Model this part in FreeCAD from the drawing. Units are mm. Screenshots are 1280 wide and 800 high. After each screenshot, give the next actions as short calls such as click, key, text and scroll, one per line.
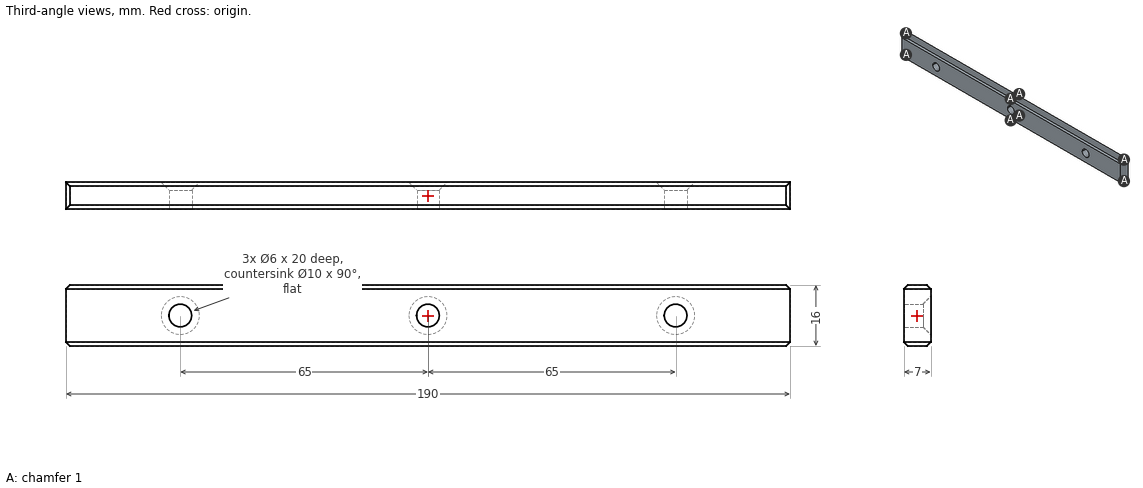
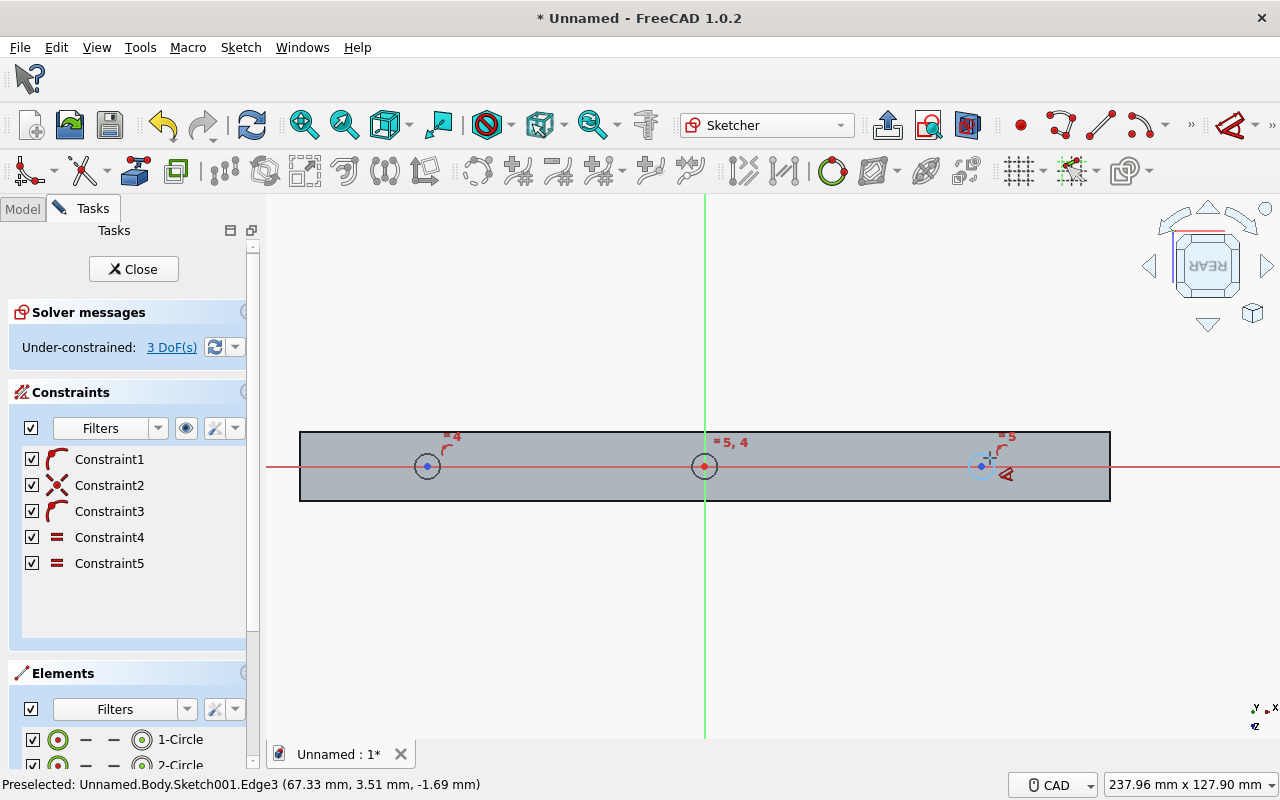
scroll(436, 458, up, 3)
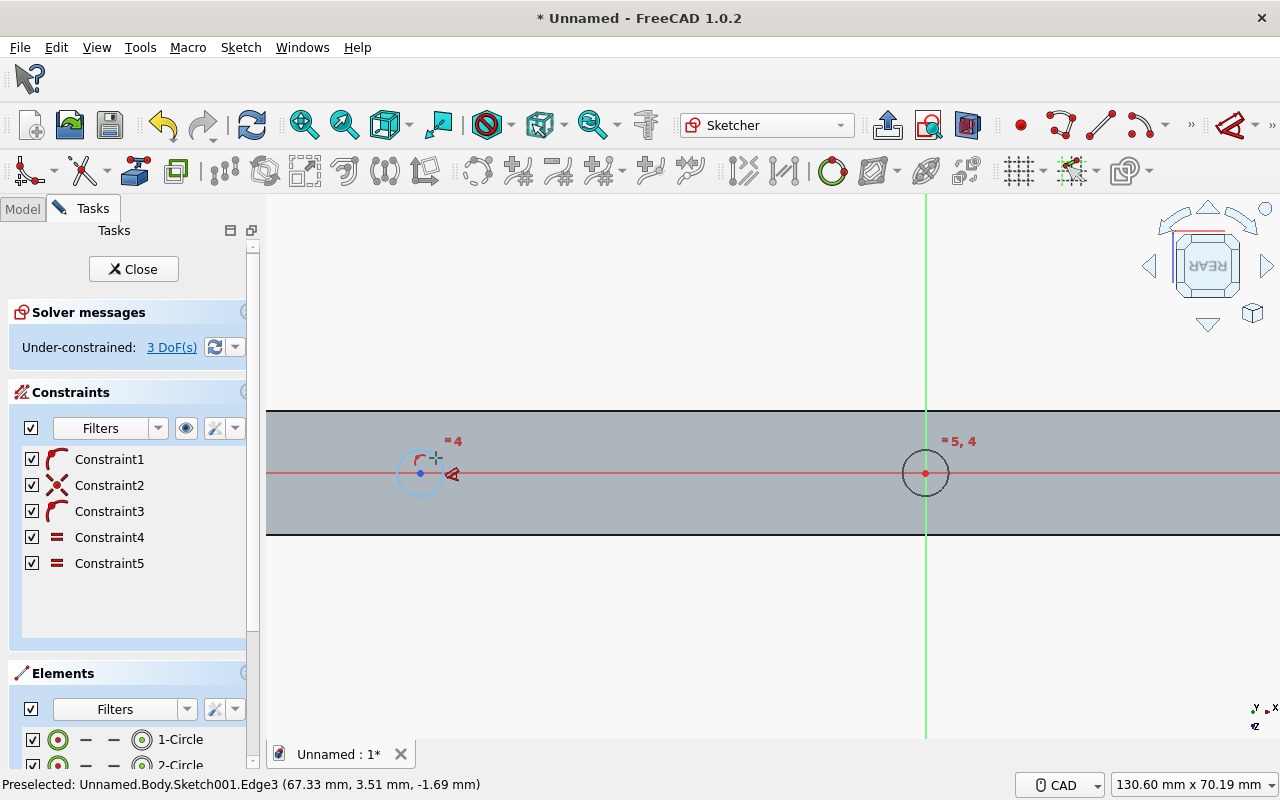
click(437, 457)
click(460, 435)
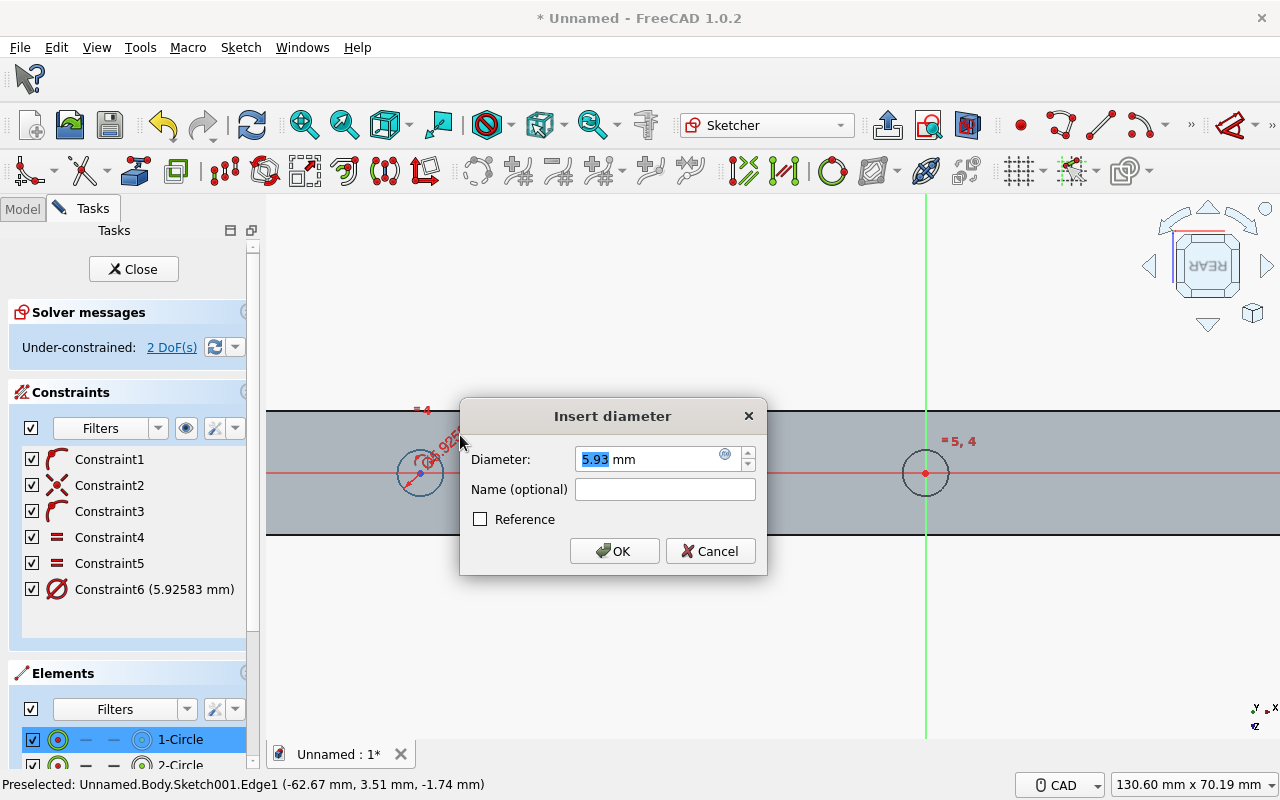
text(6)
key(Return)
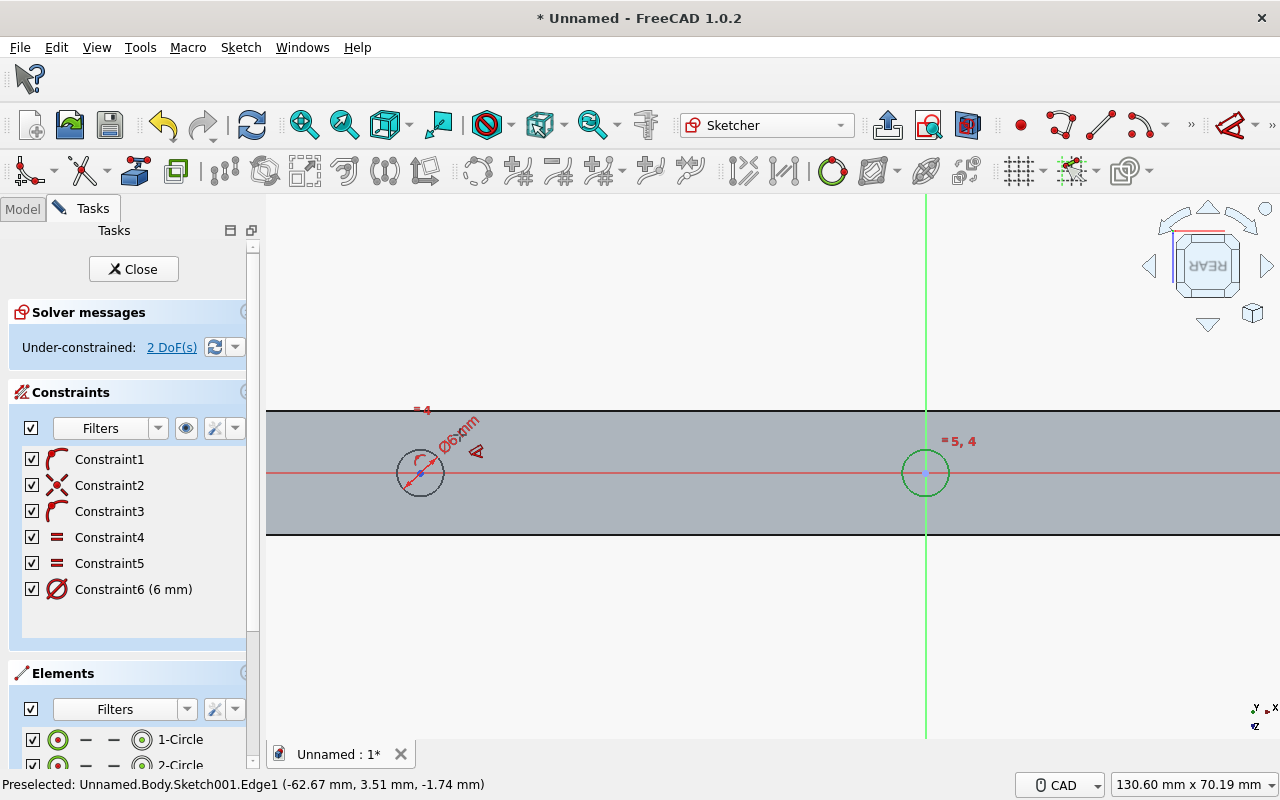
click(420, 473)
click(673, 507)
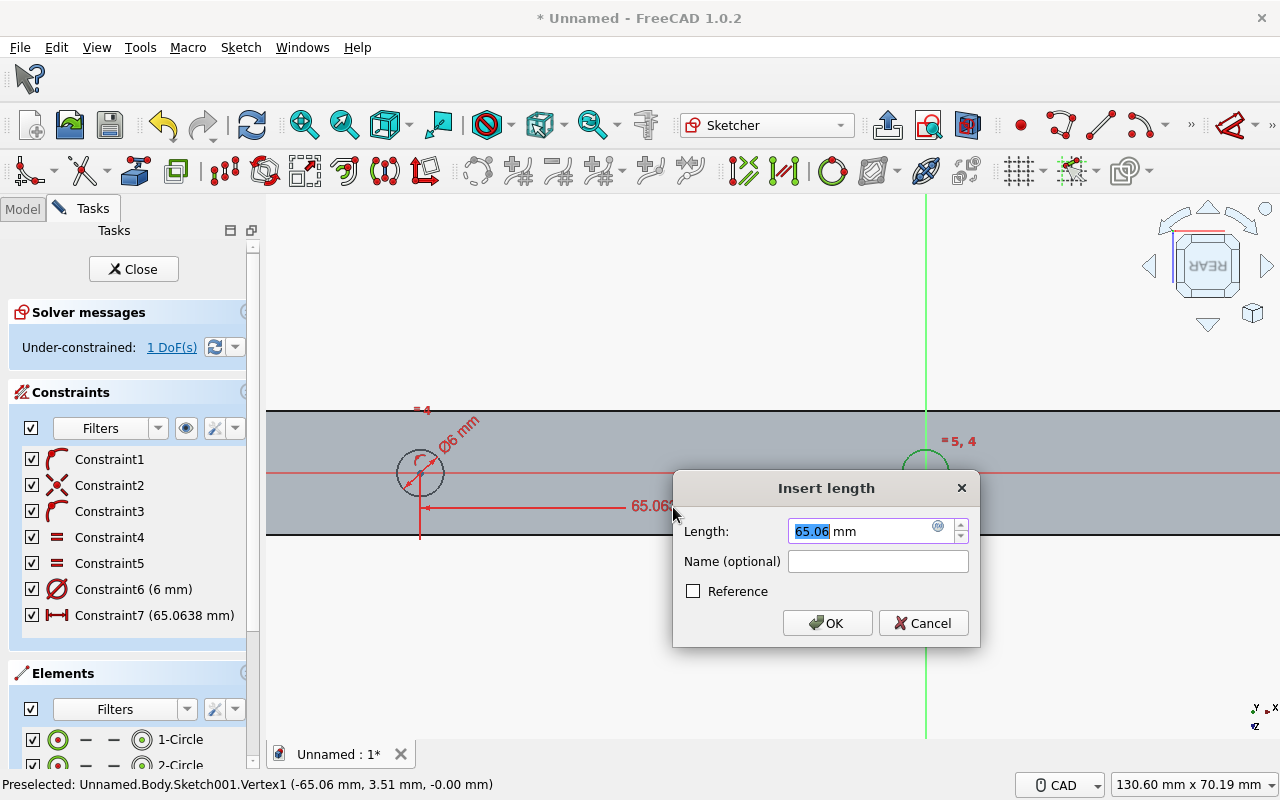
text(65)
key(Return)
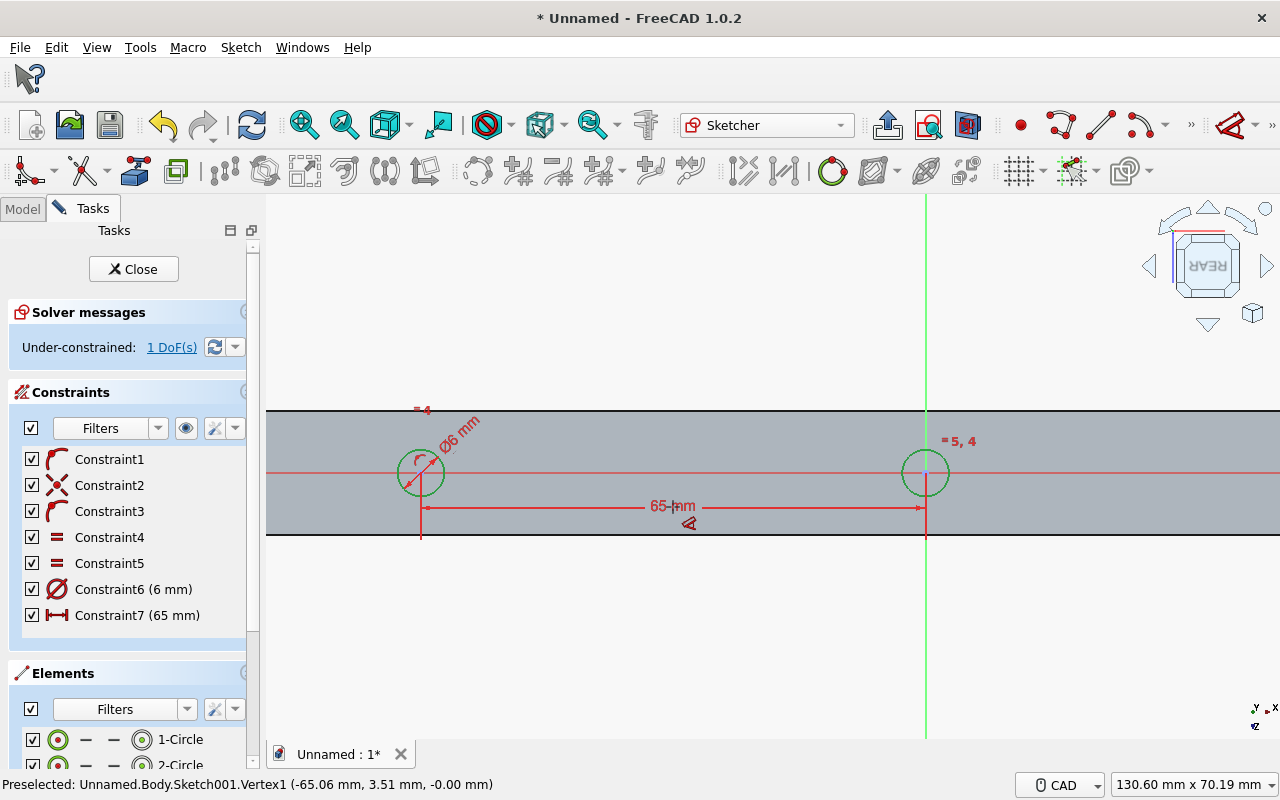
scroll(436, 458, down, 3)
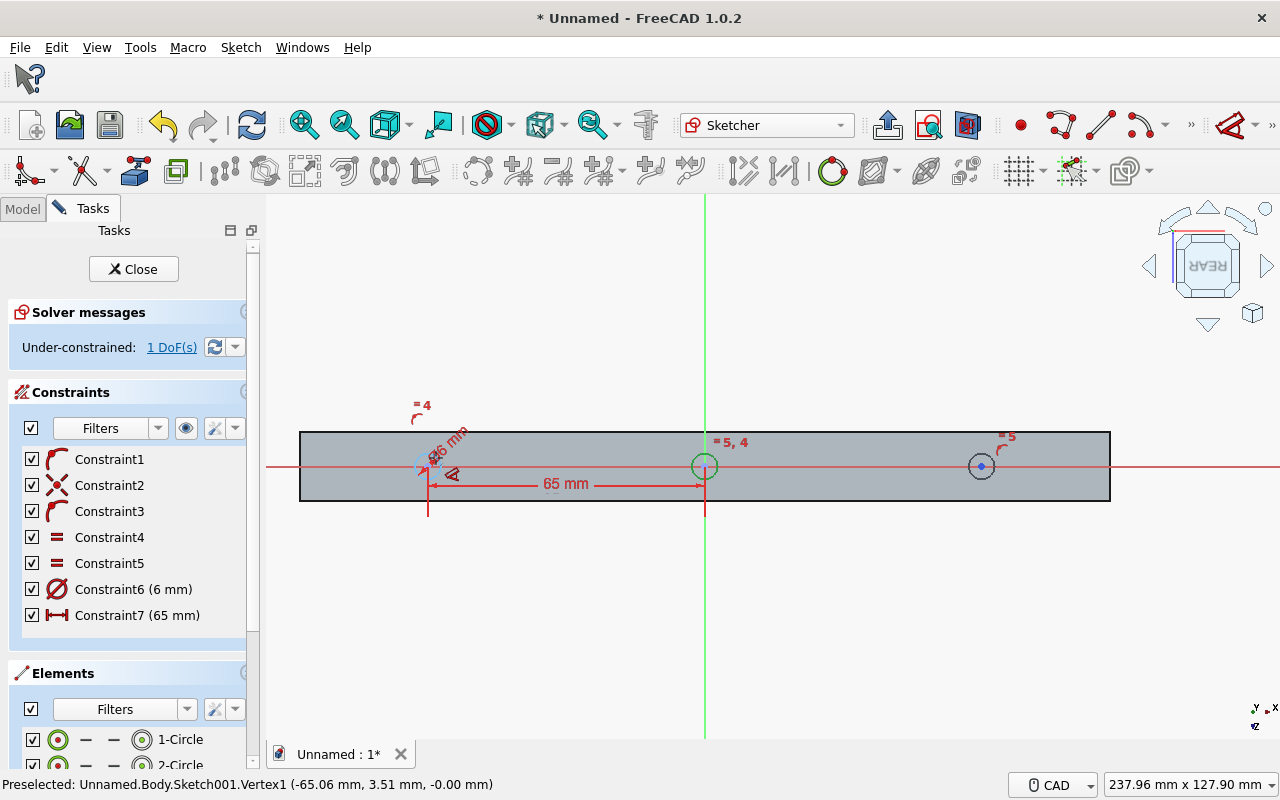
click(982, 466)
click(843, 500)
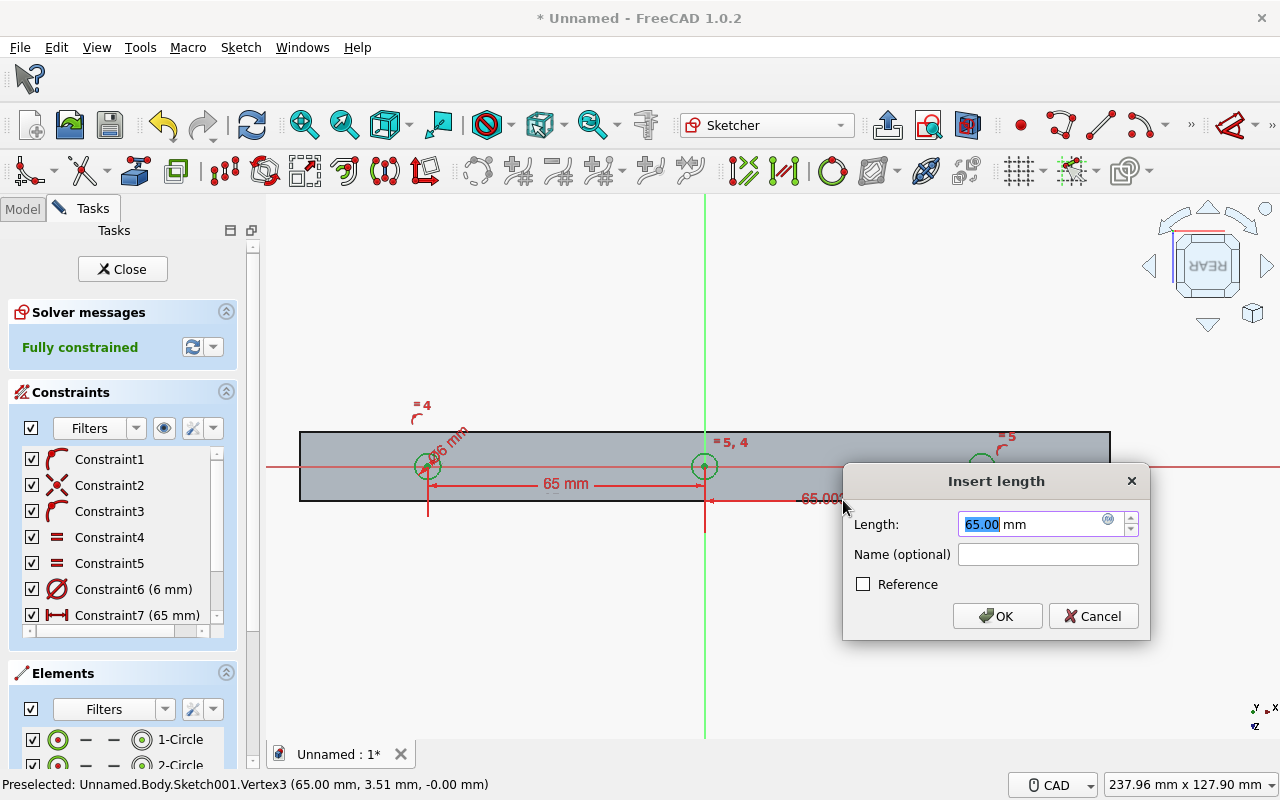
text(65)
key(Return)
key(Escape)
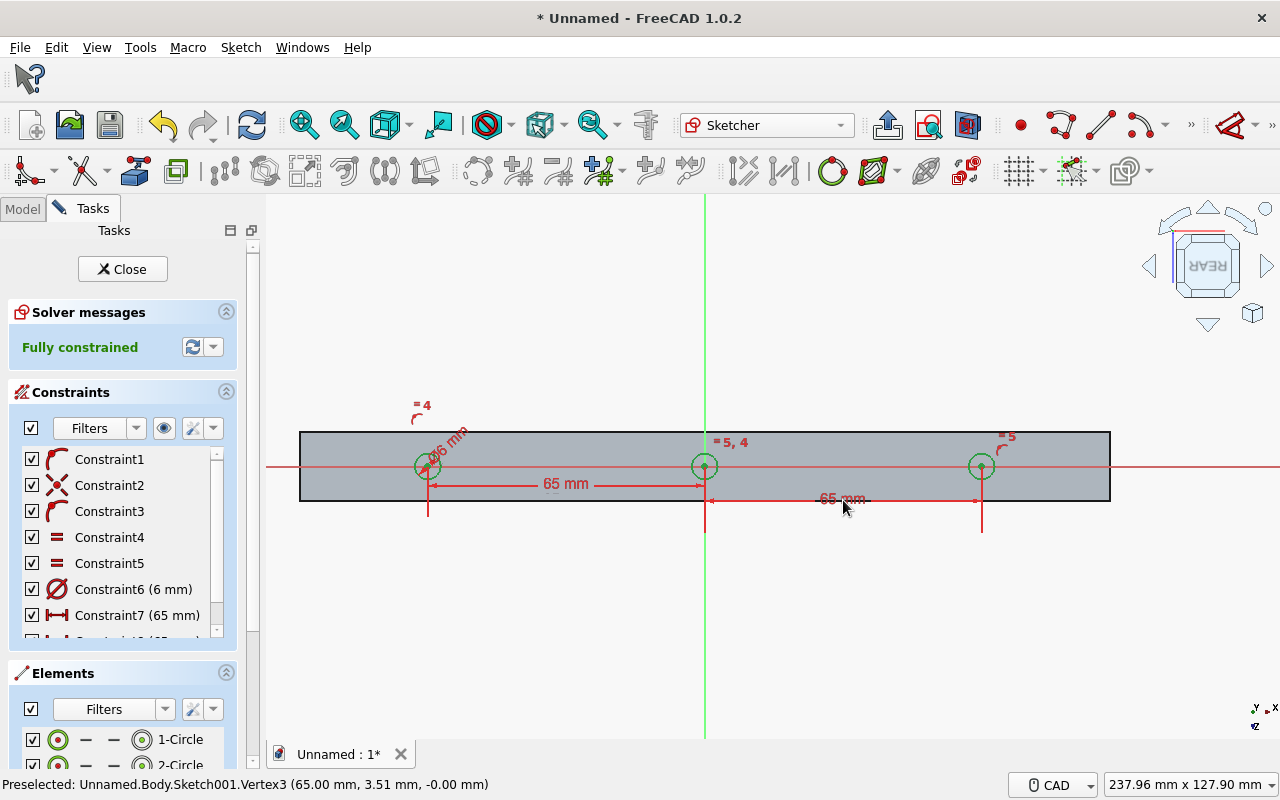
click(123, 269)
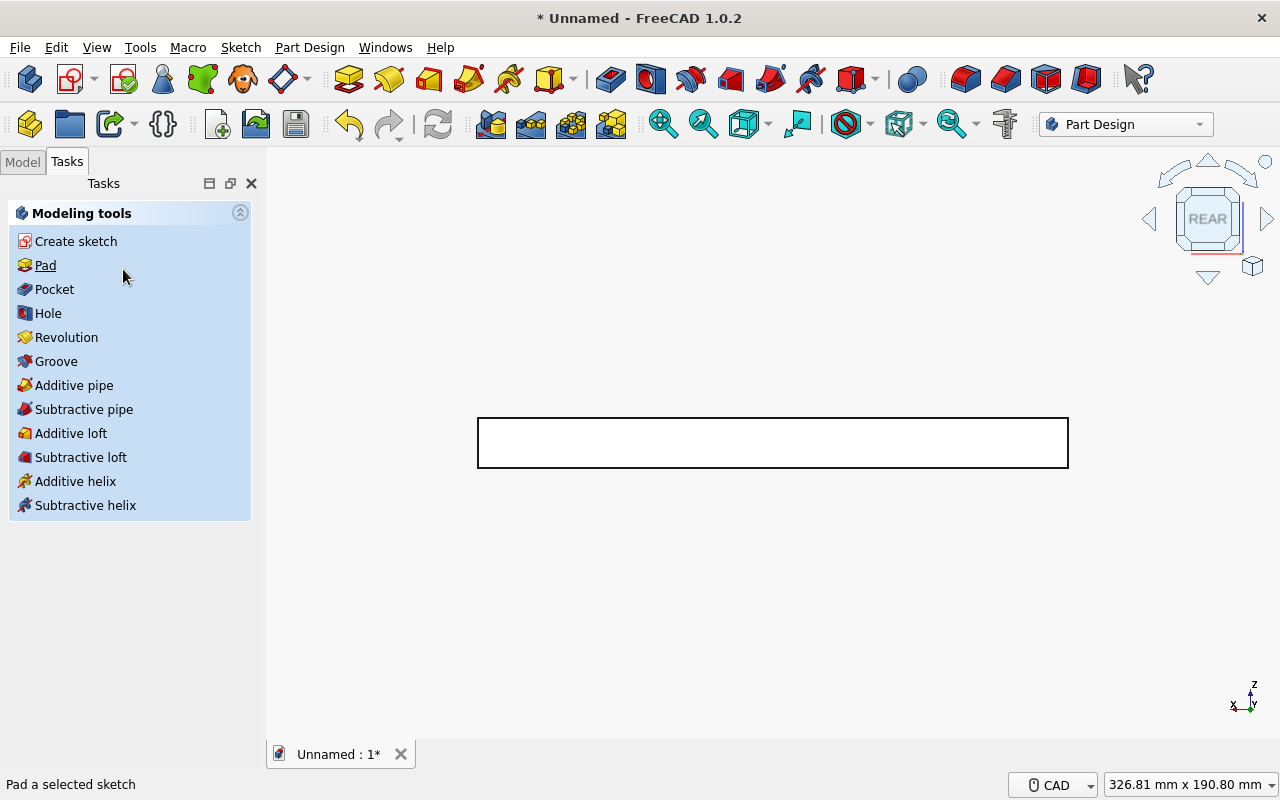
click(652, 80)